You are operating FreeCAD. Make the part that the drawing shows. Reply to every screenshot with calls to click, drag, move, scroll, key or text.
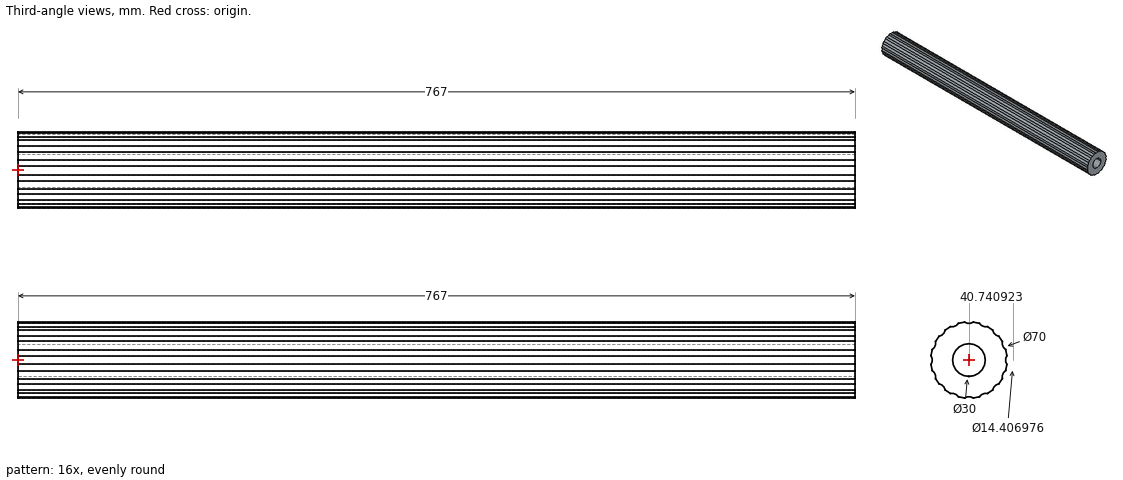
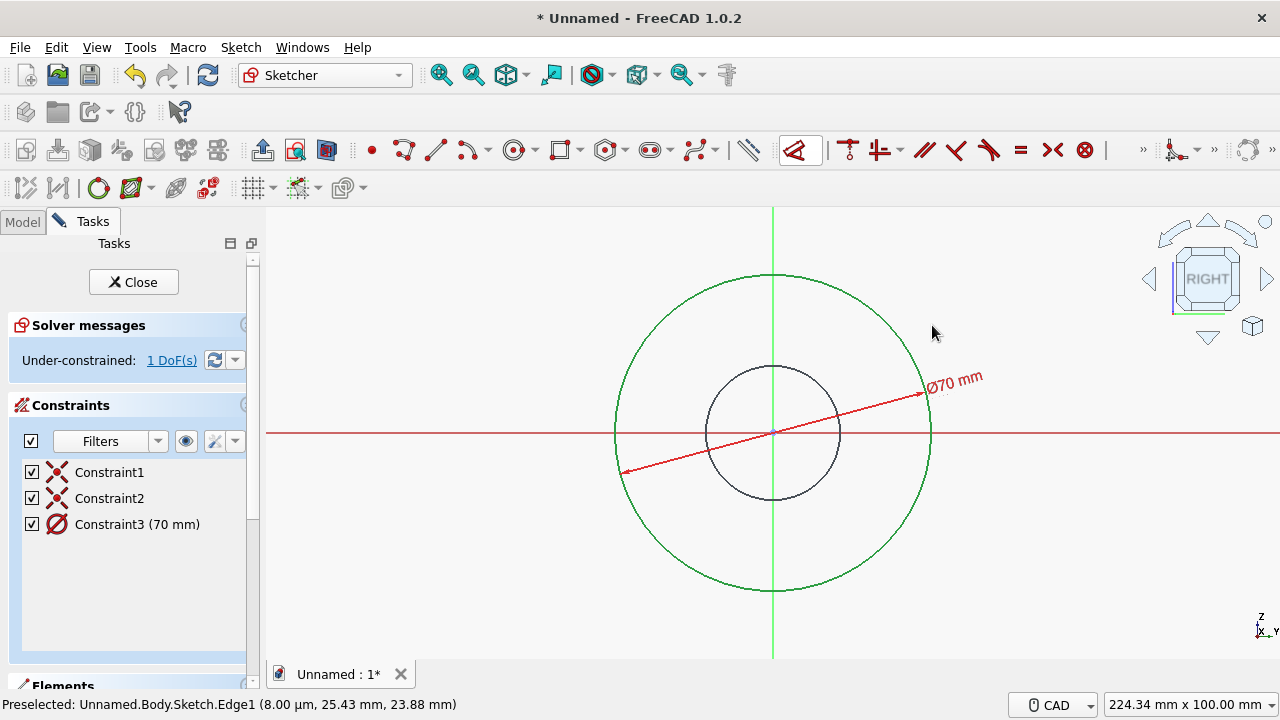
click(820, 385)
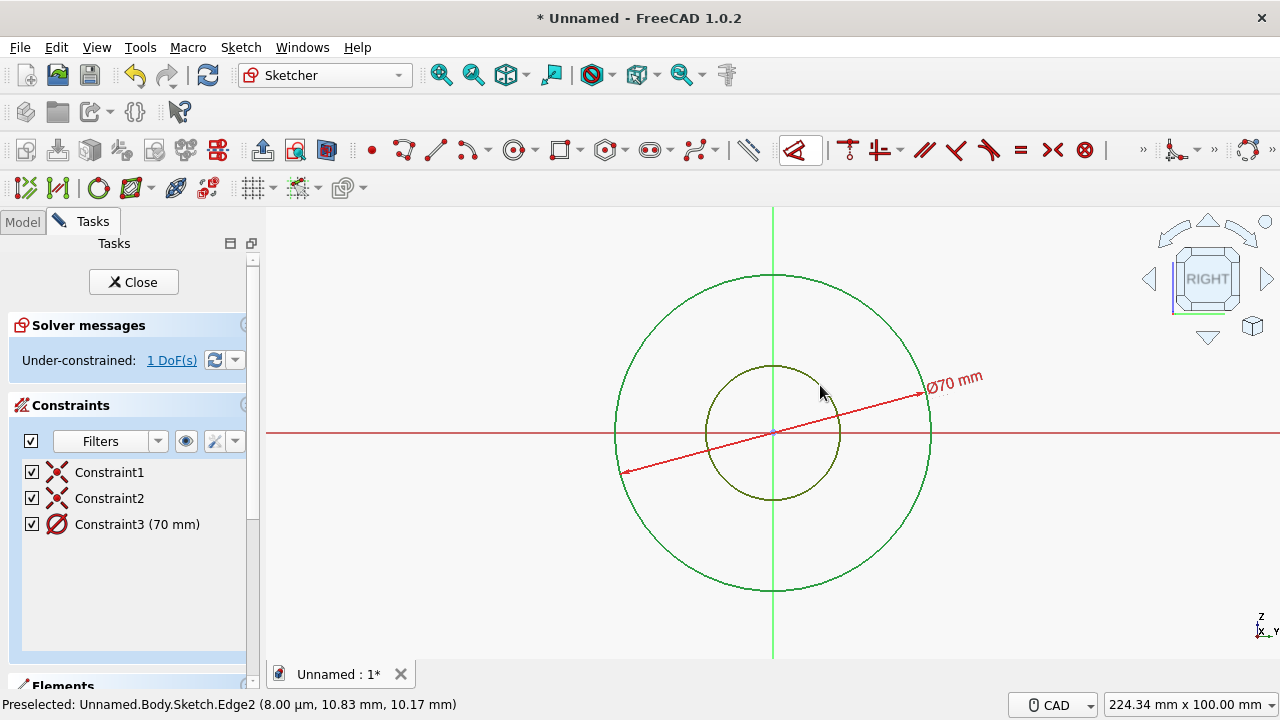
key(k)
key(o)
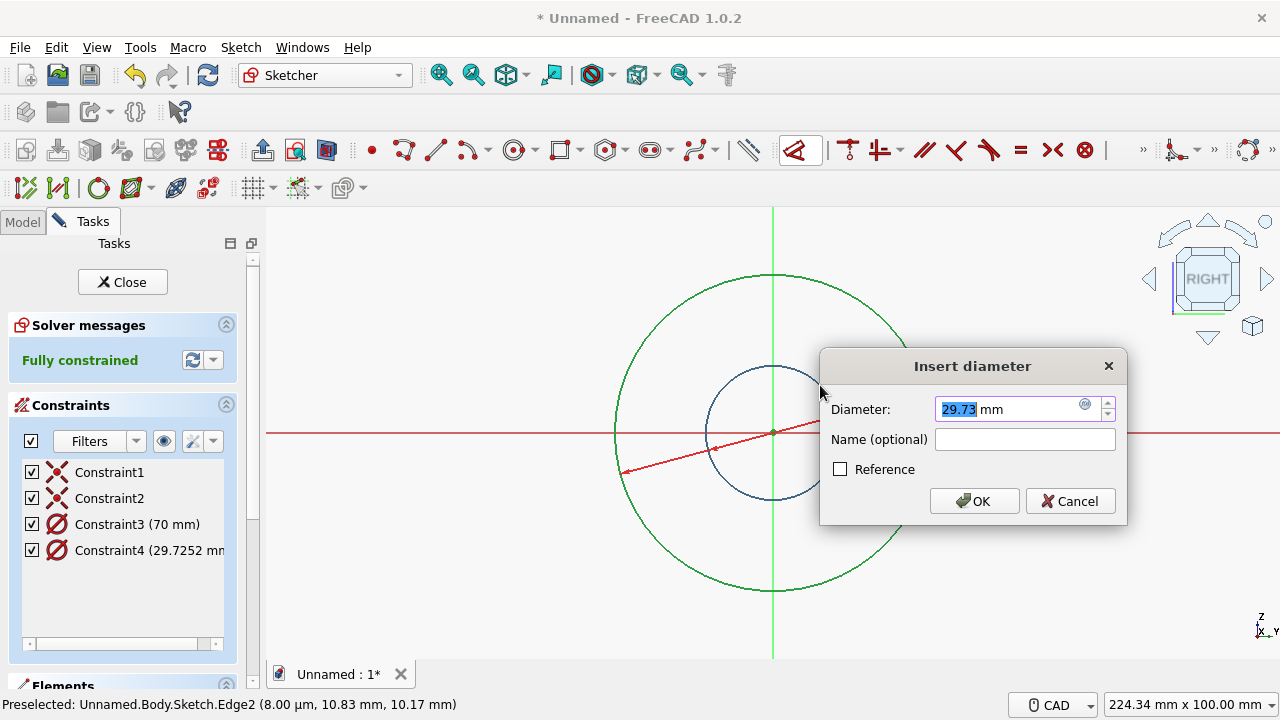
text(30)
key(Return)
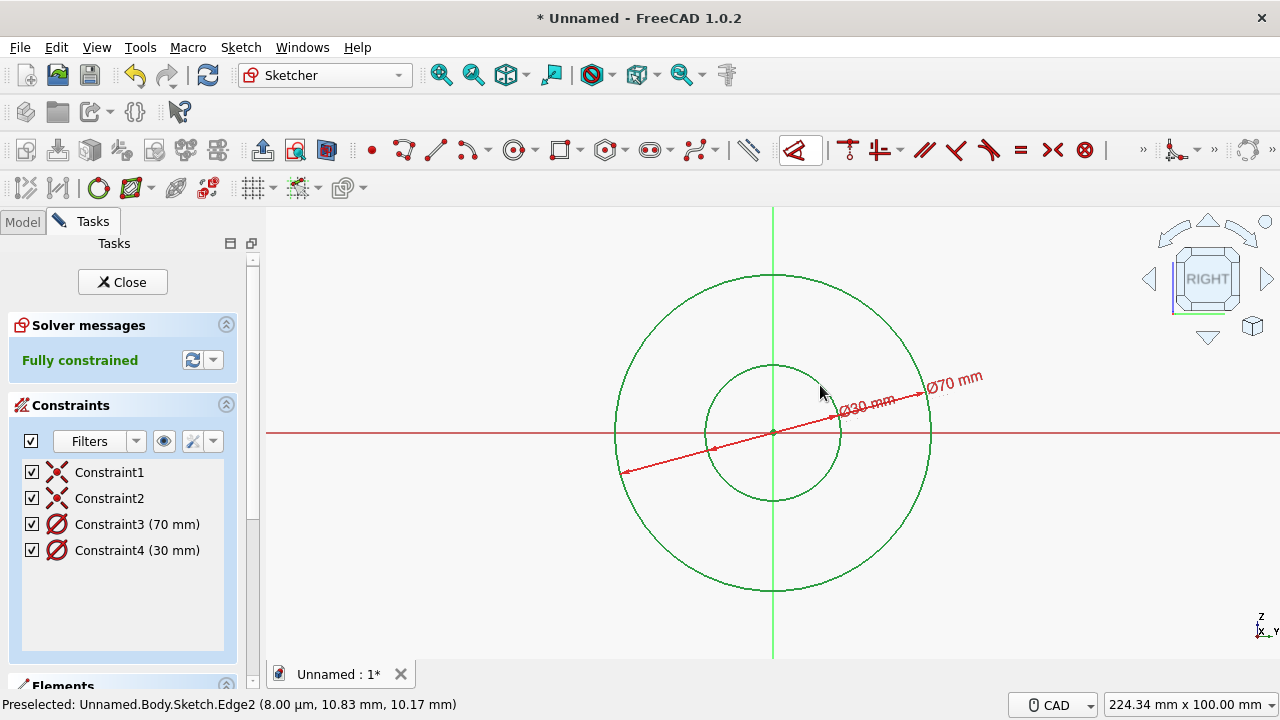
click(123, 282)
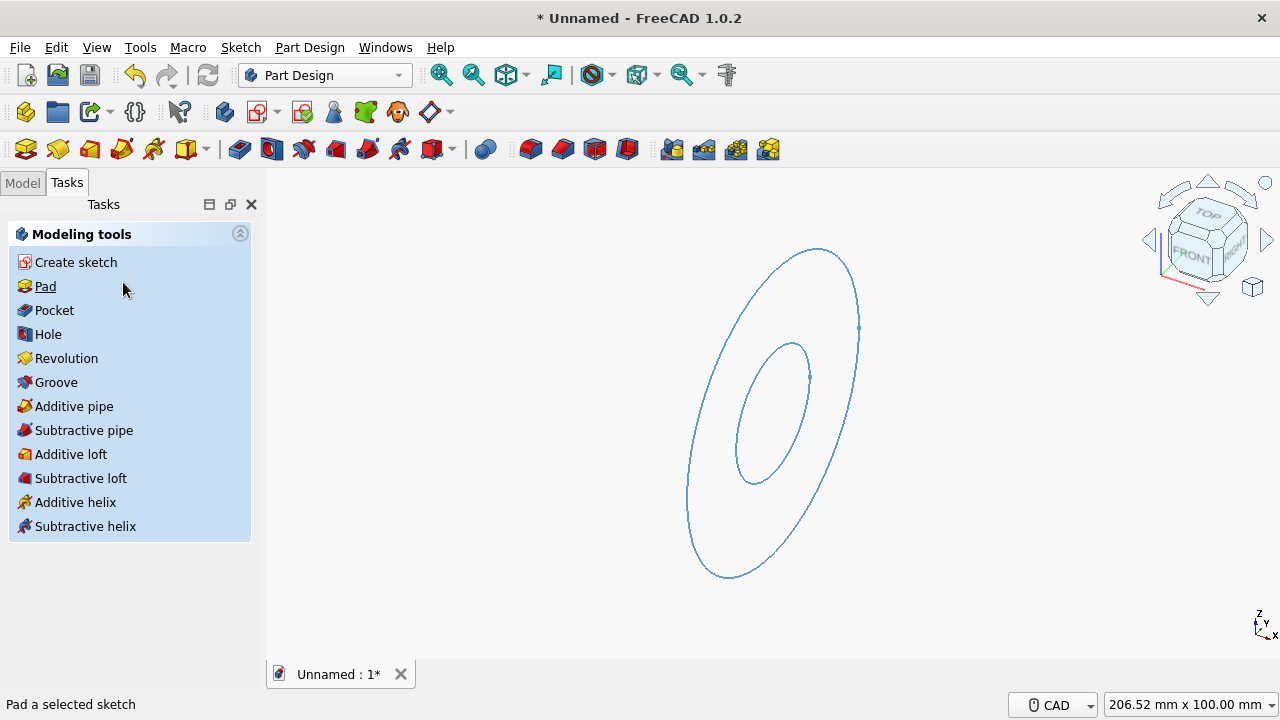
click(26, 150)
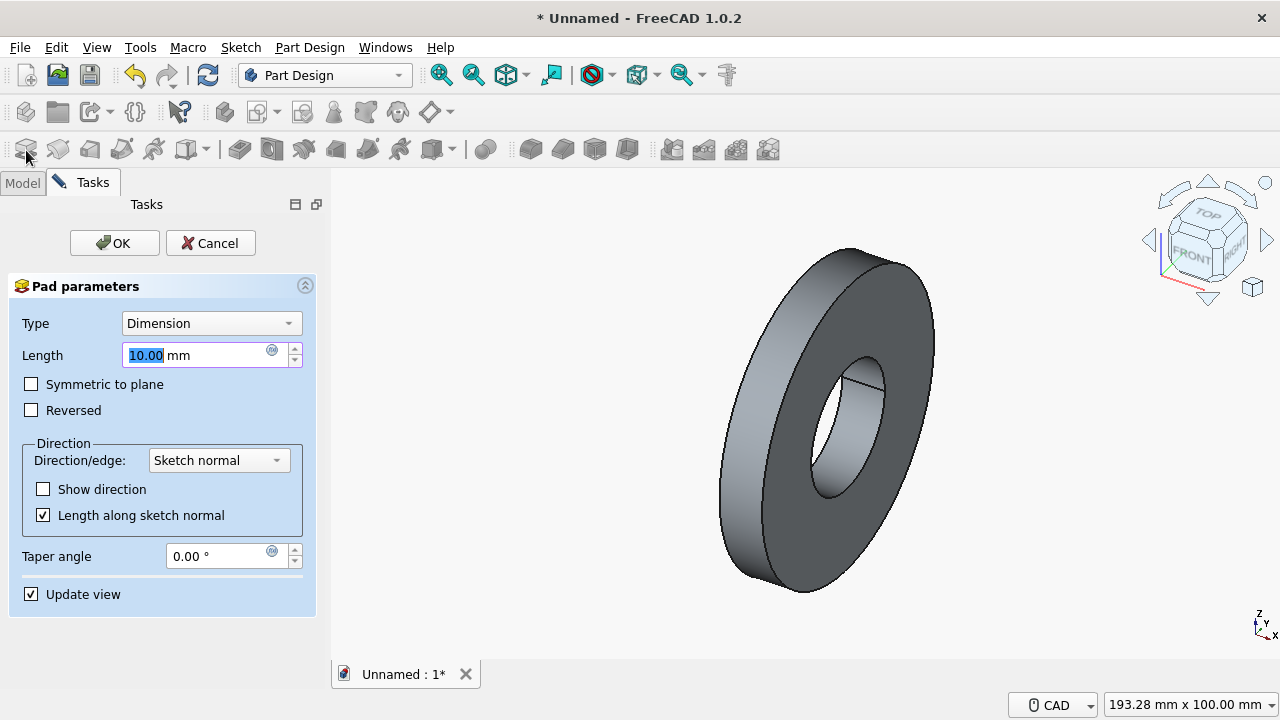
text(767)
key(Tab)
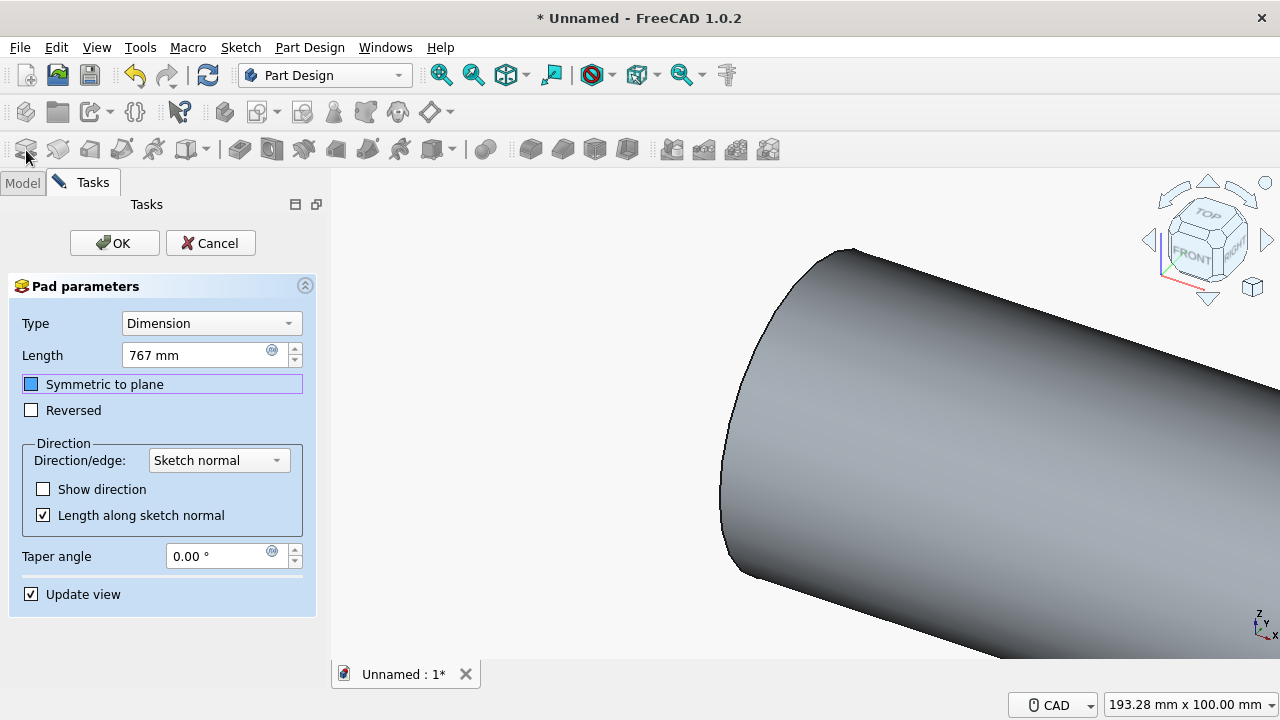
click(115, 243)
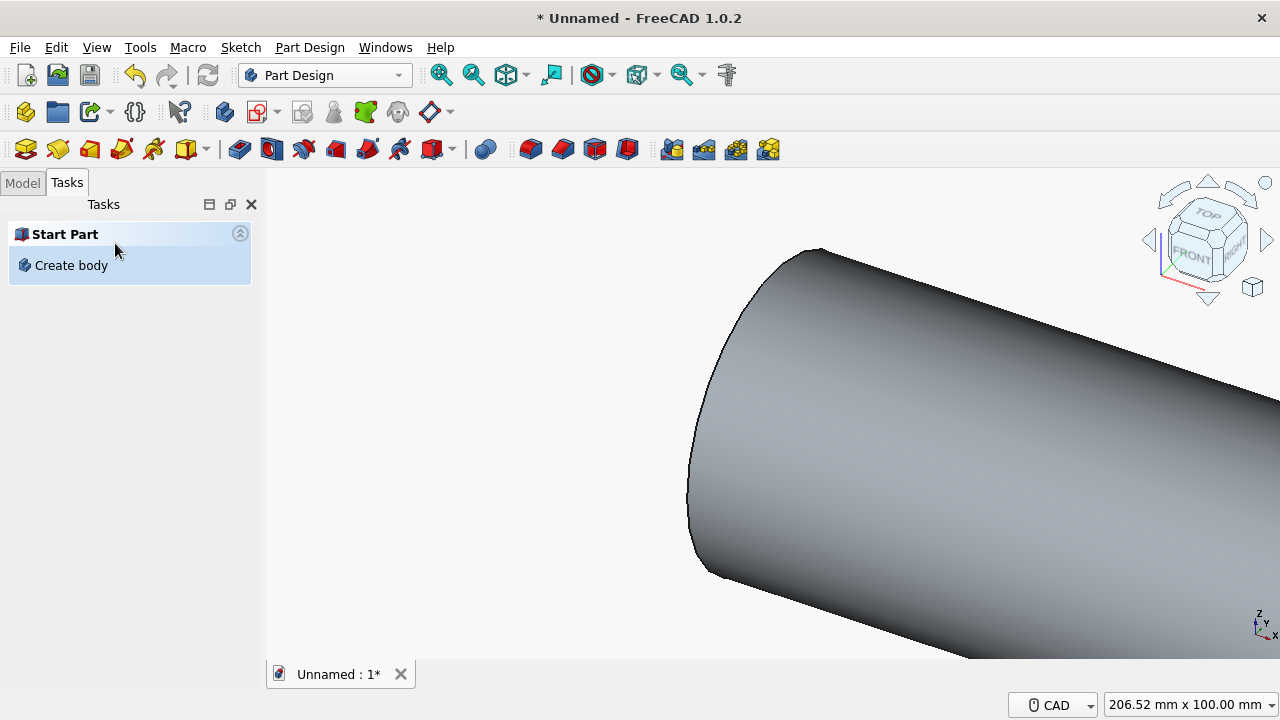
click(442, 76)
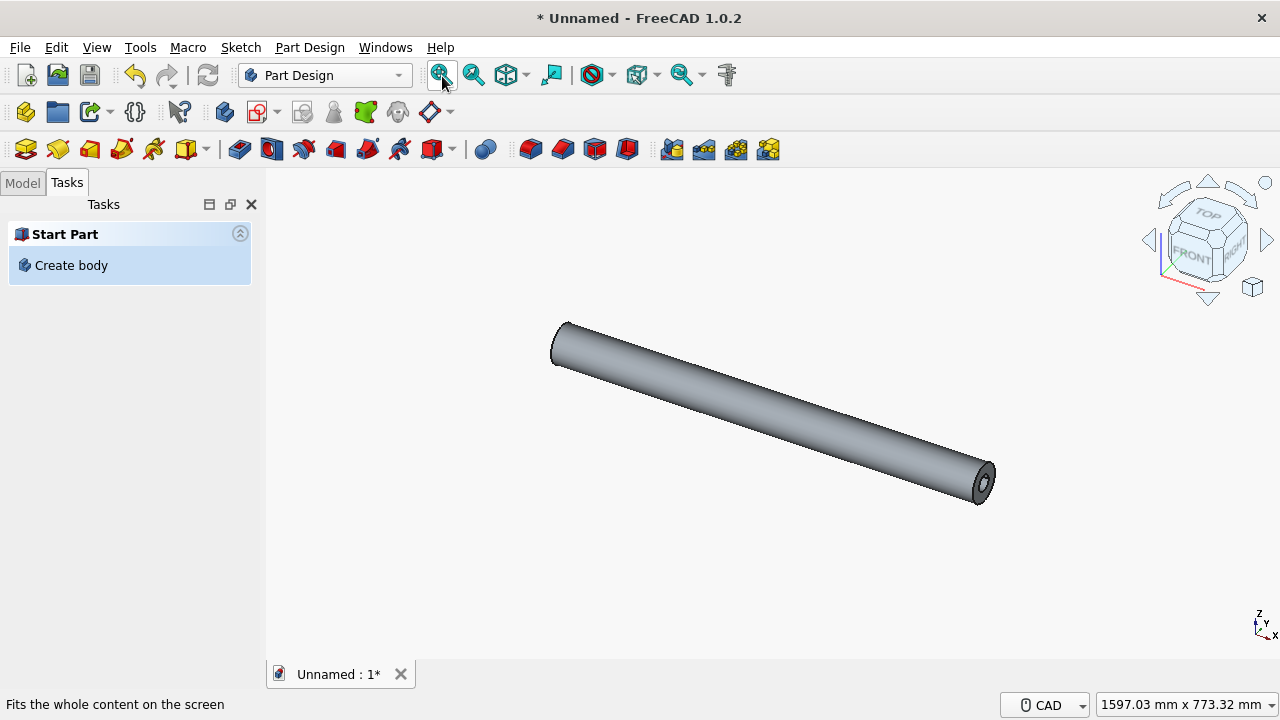
click(258, 112)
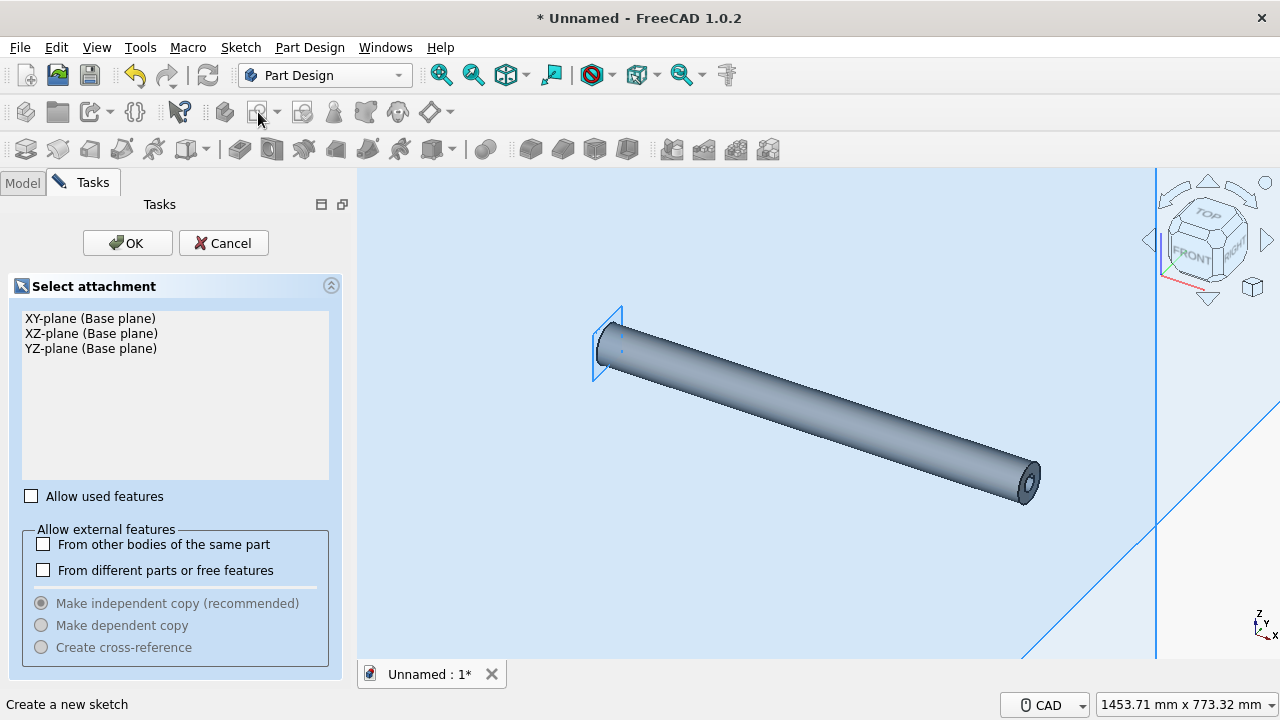
click(82, 348)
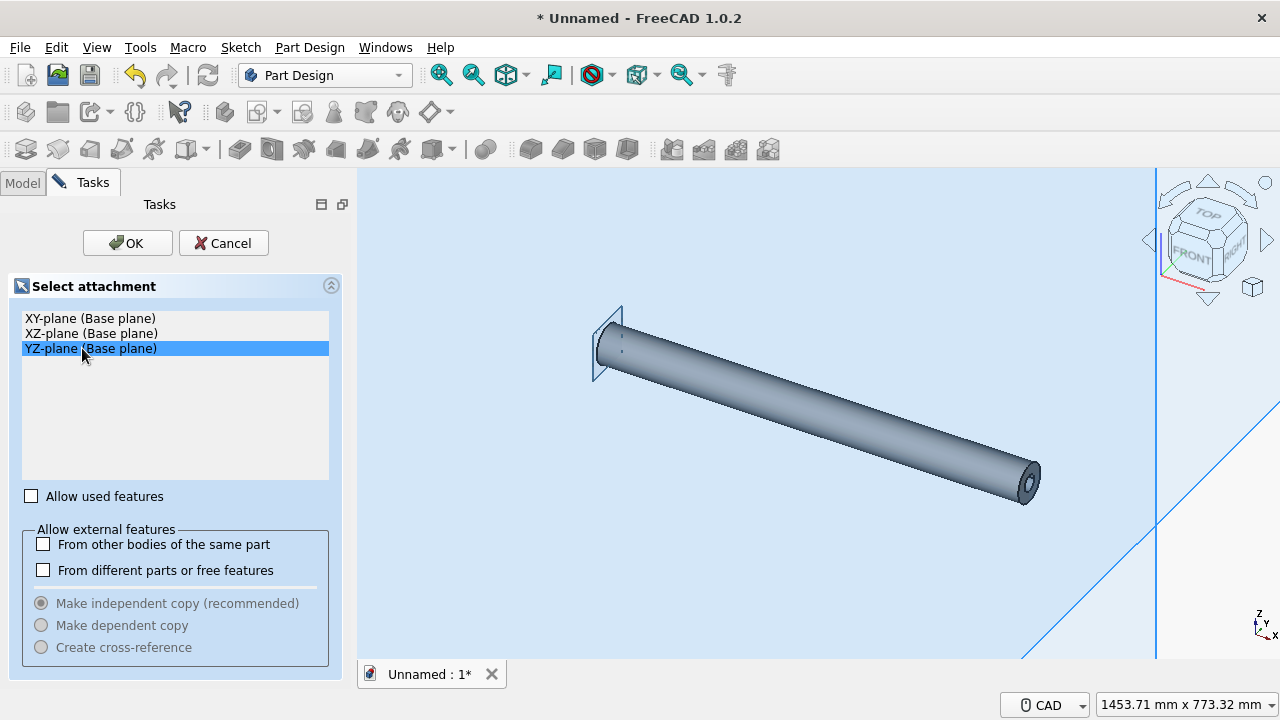
click(128, 243)